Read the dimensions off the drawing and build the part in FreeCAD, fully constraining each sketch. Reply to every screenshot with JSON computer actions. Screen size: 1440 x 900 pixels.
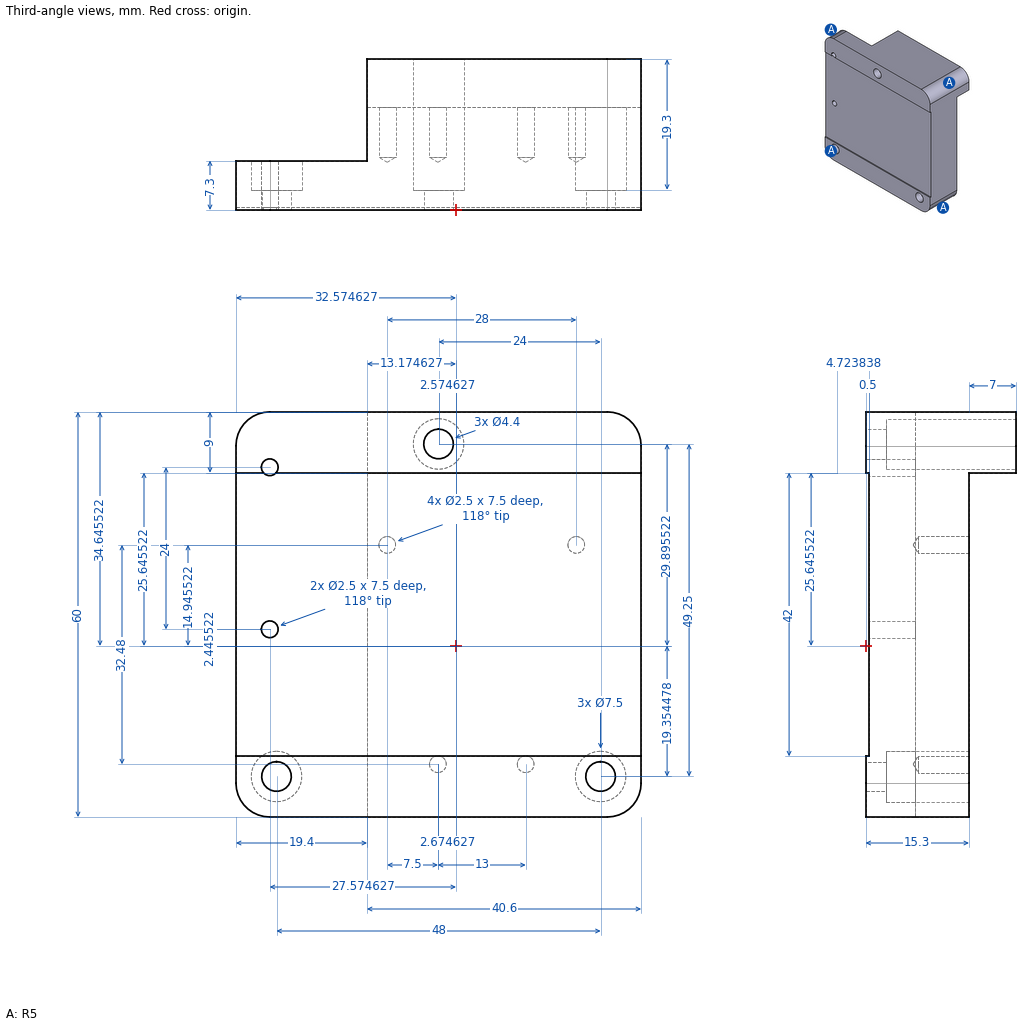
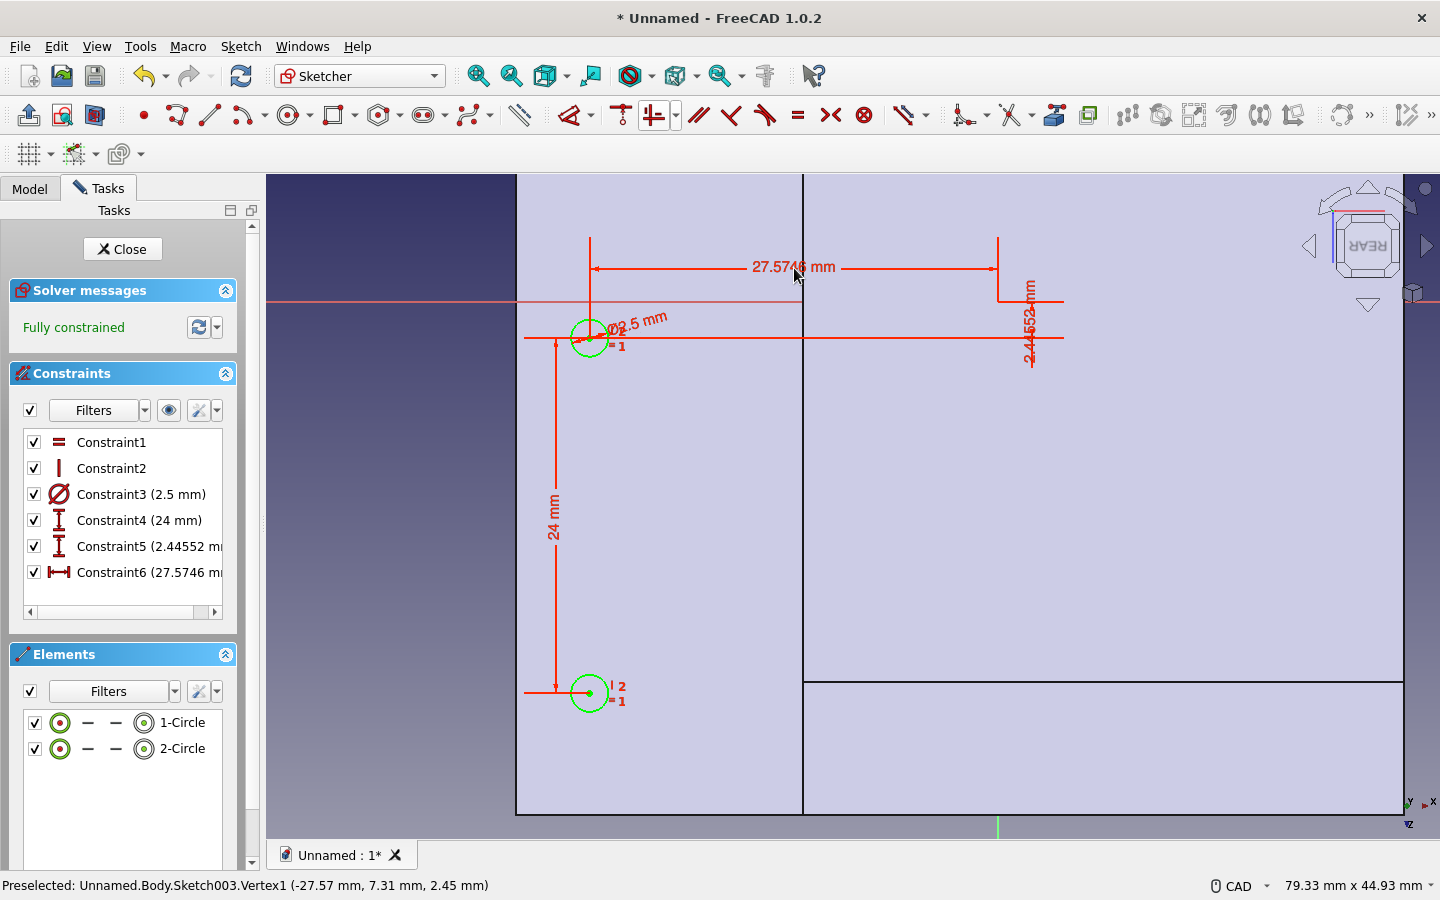
{"action": "left_click", "coordinate": [123, 249]}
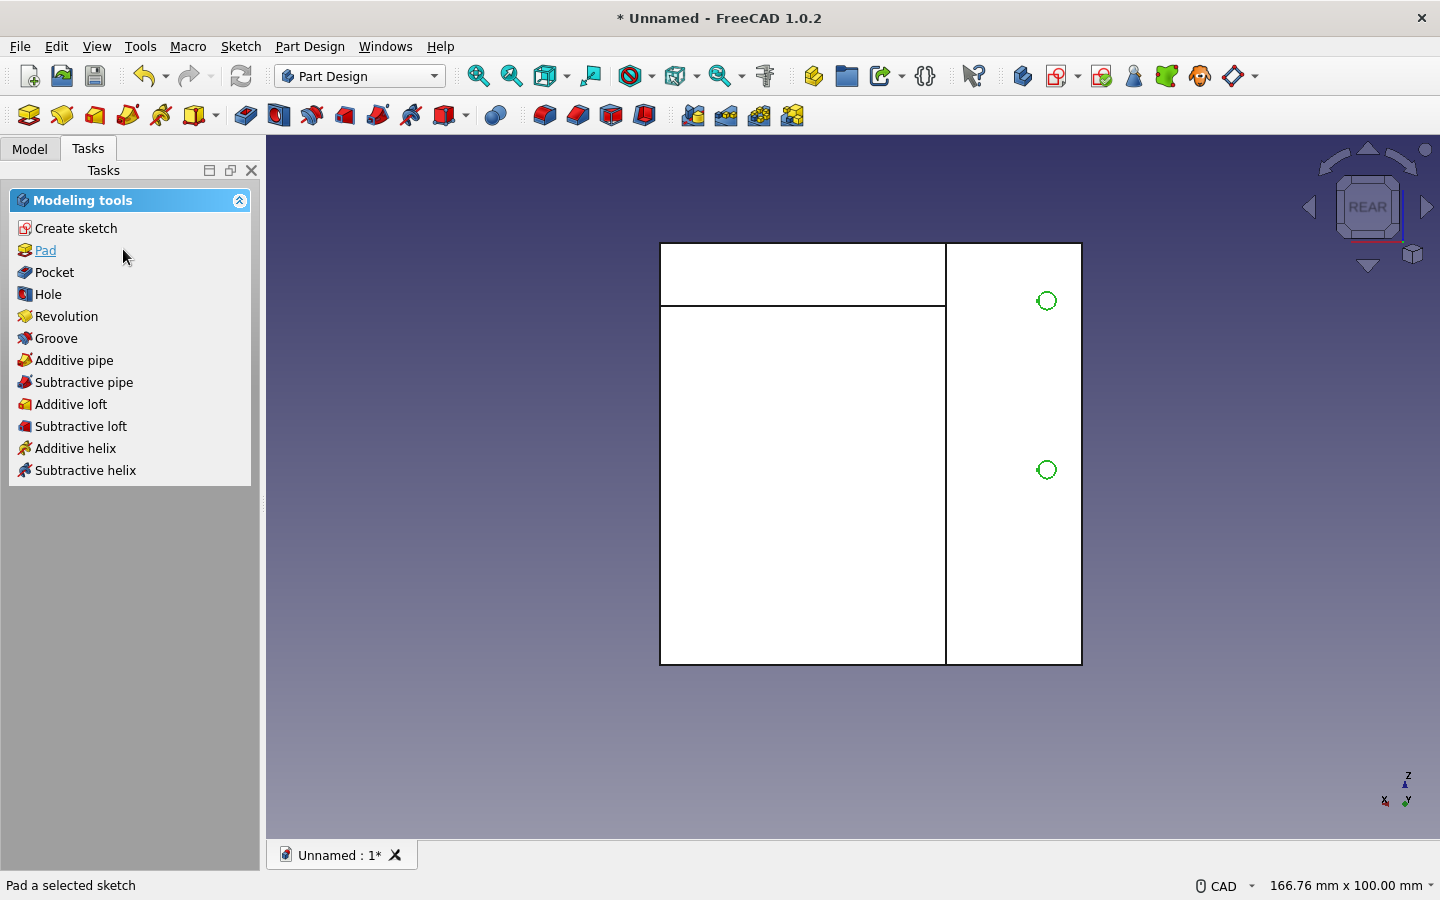
{"action": "left_click", "coordinate": [279, 116]}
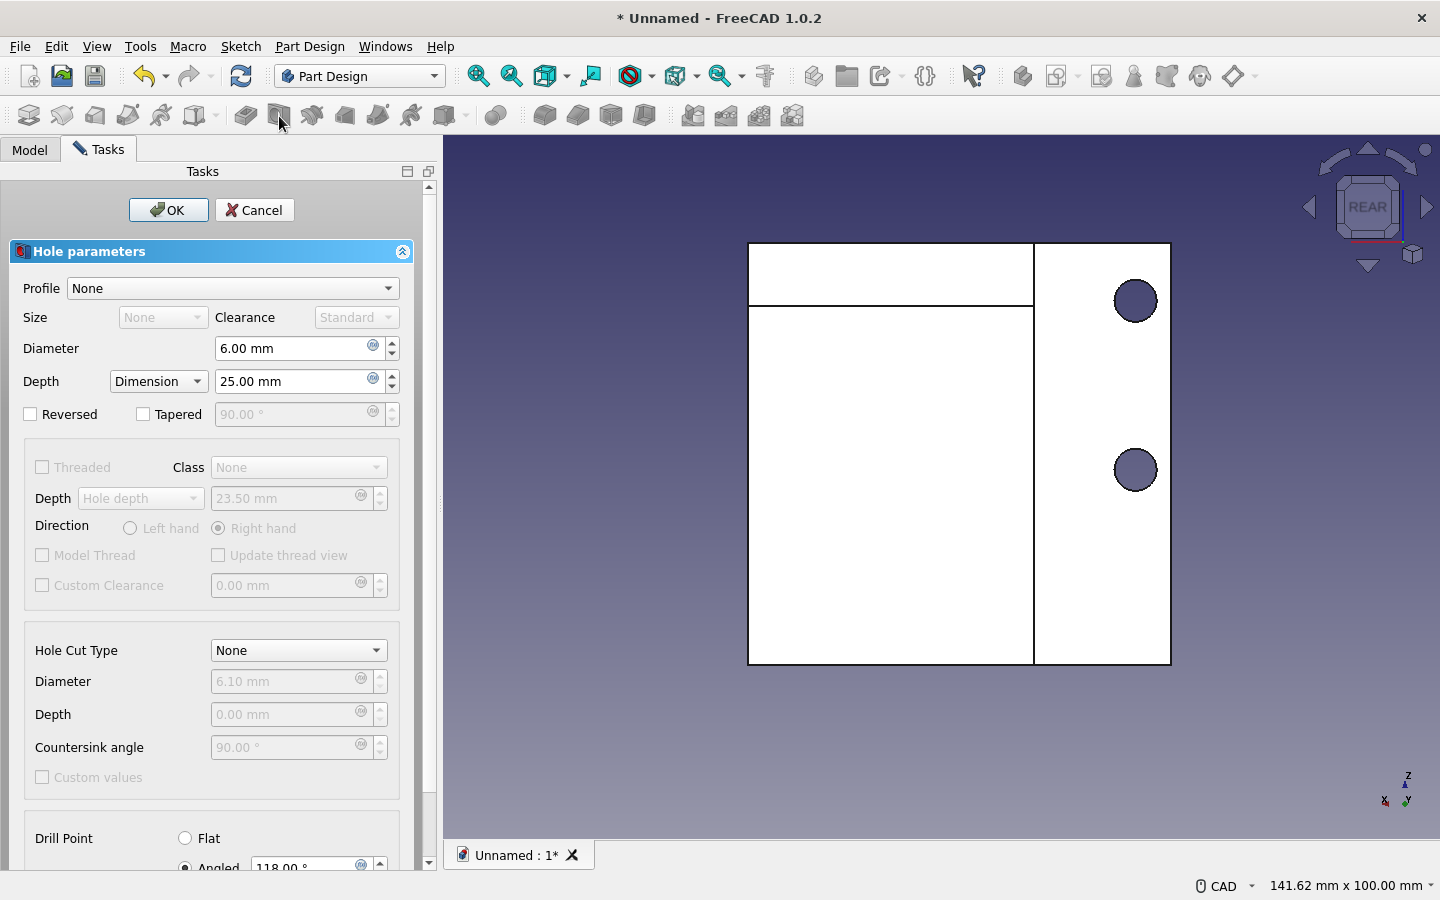
{"action": "triple_click", "coordinate": [300, 348]}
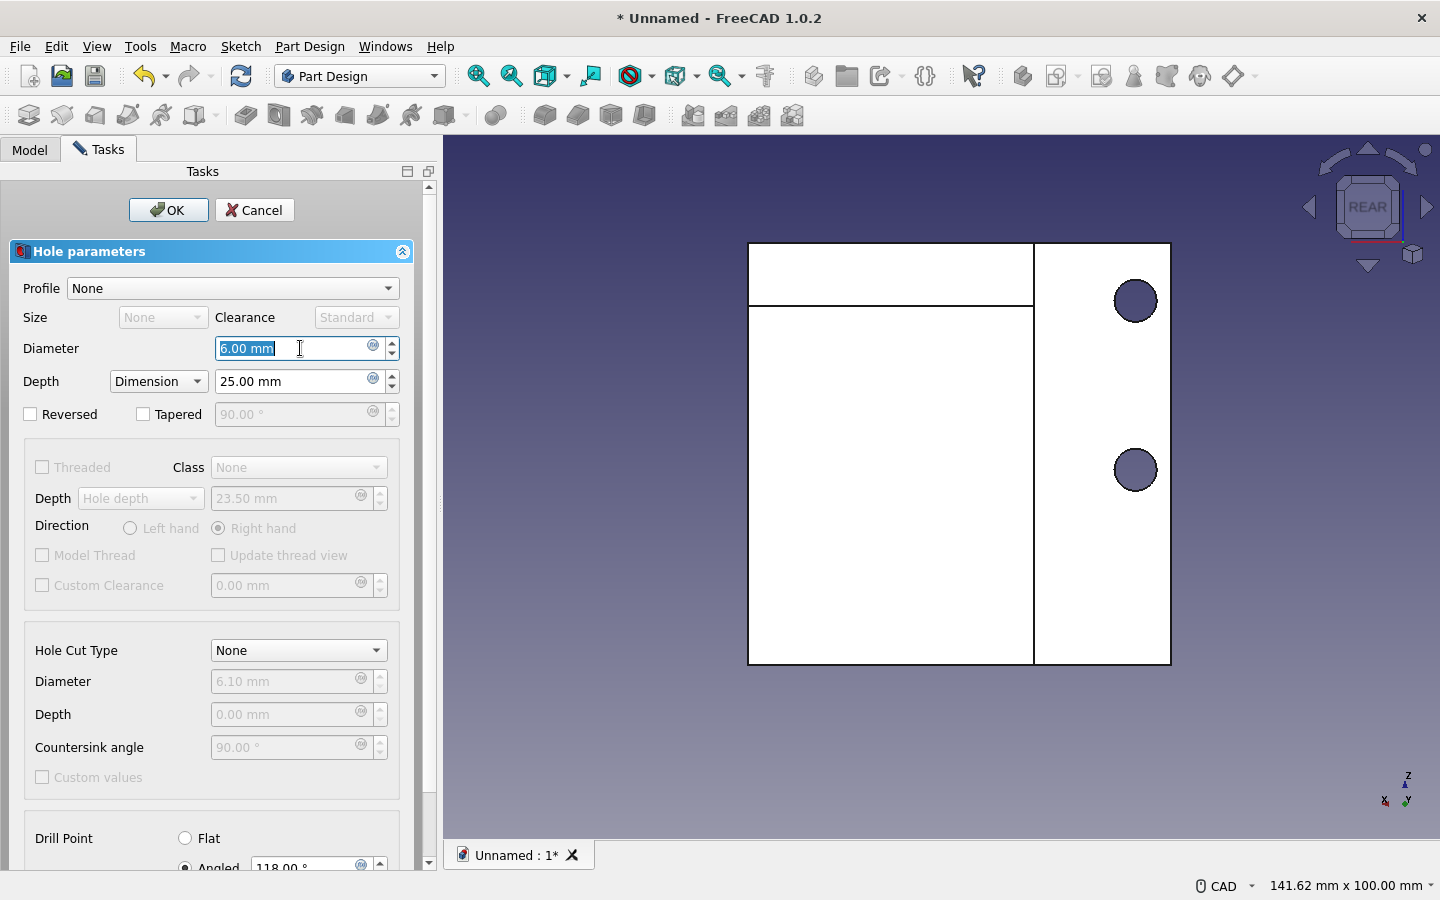
{"action": "type", "text": "2.5"}
{"action": "key", "text": "Tab"}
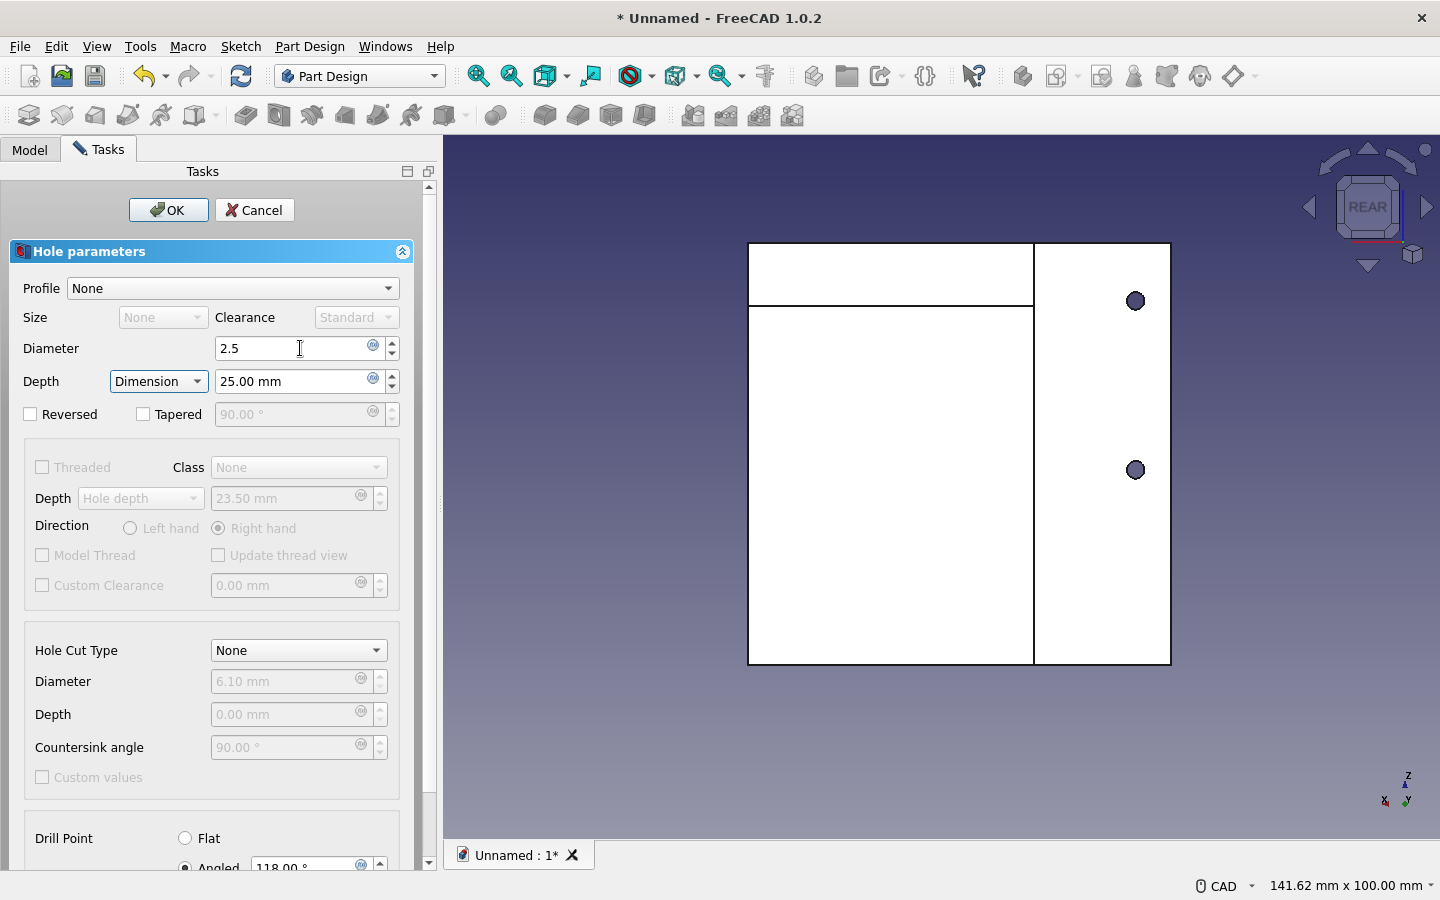
{"action": "triple_click", "coordinate": [300, 382]}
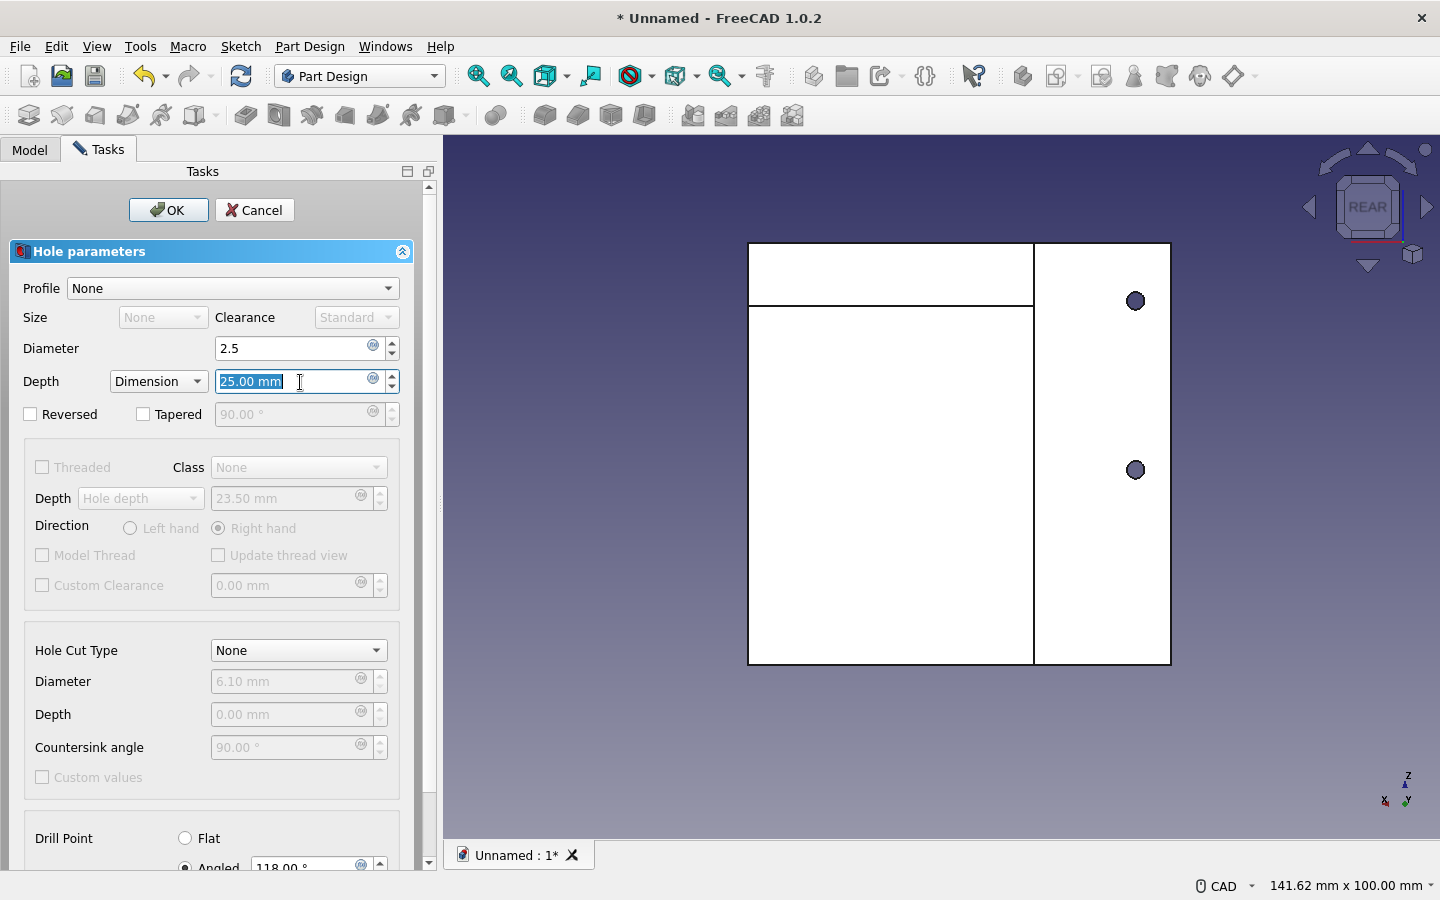
{"action": "type", "text": "7.5"}
{"action": "key", "text": "Tab"}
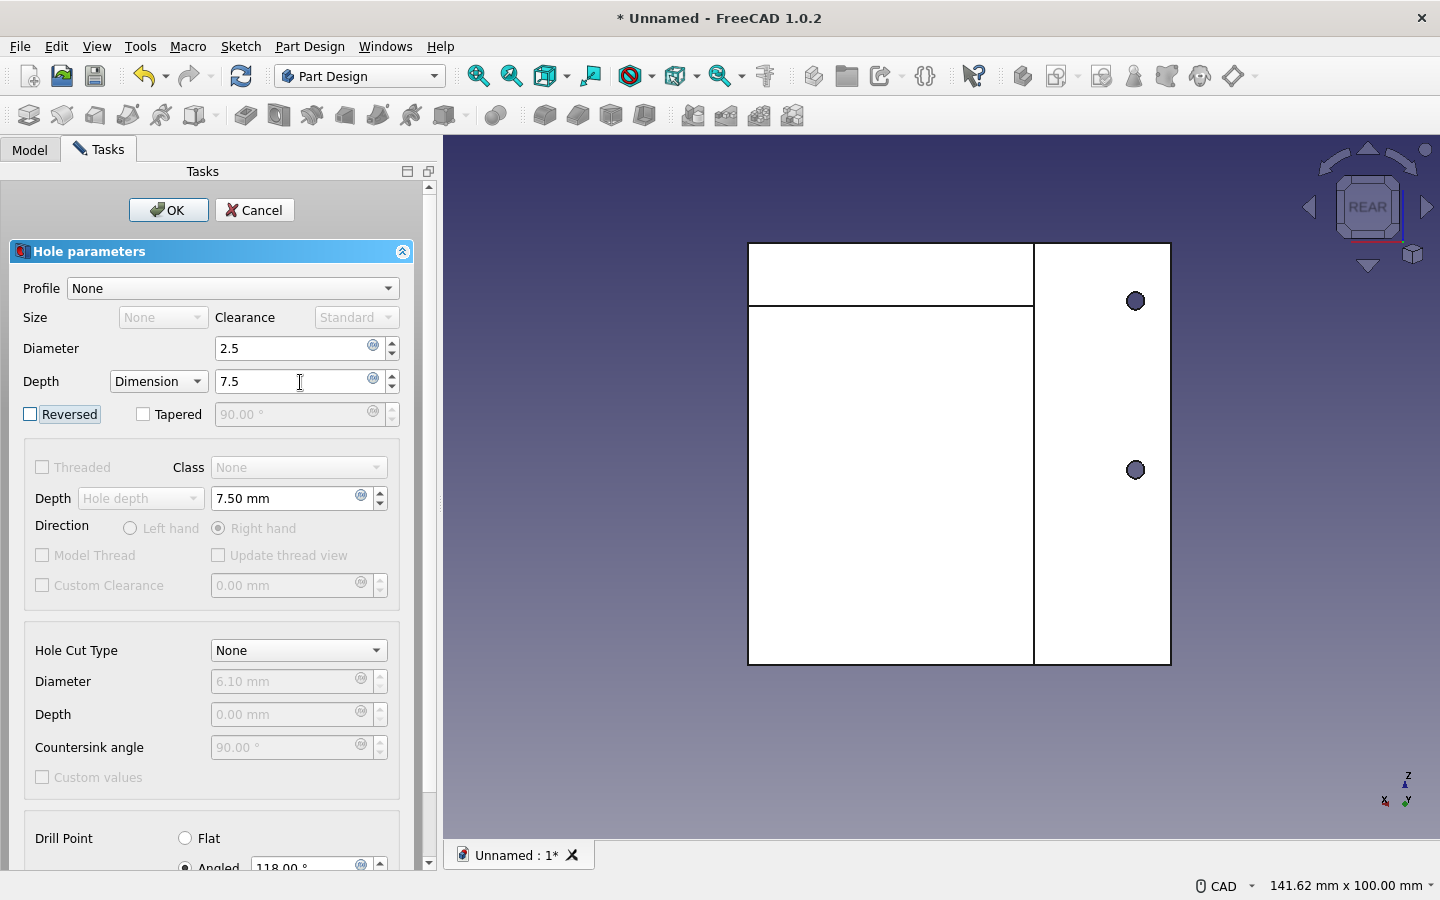
{"action": "left_click", "coordinate": [169, 210]}